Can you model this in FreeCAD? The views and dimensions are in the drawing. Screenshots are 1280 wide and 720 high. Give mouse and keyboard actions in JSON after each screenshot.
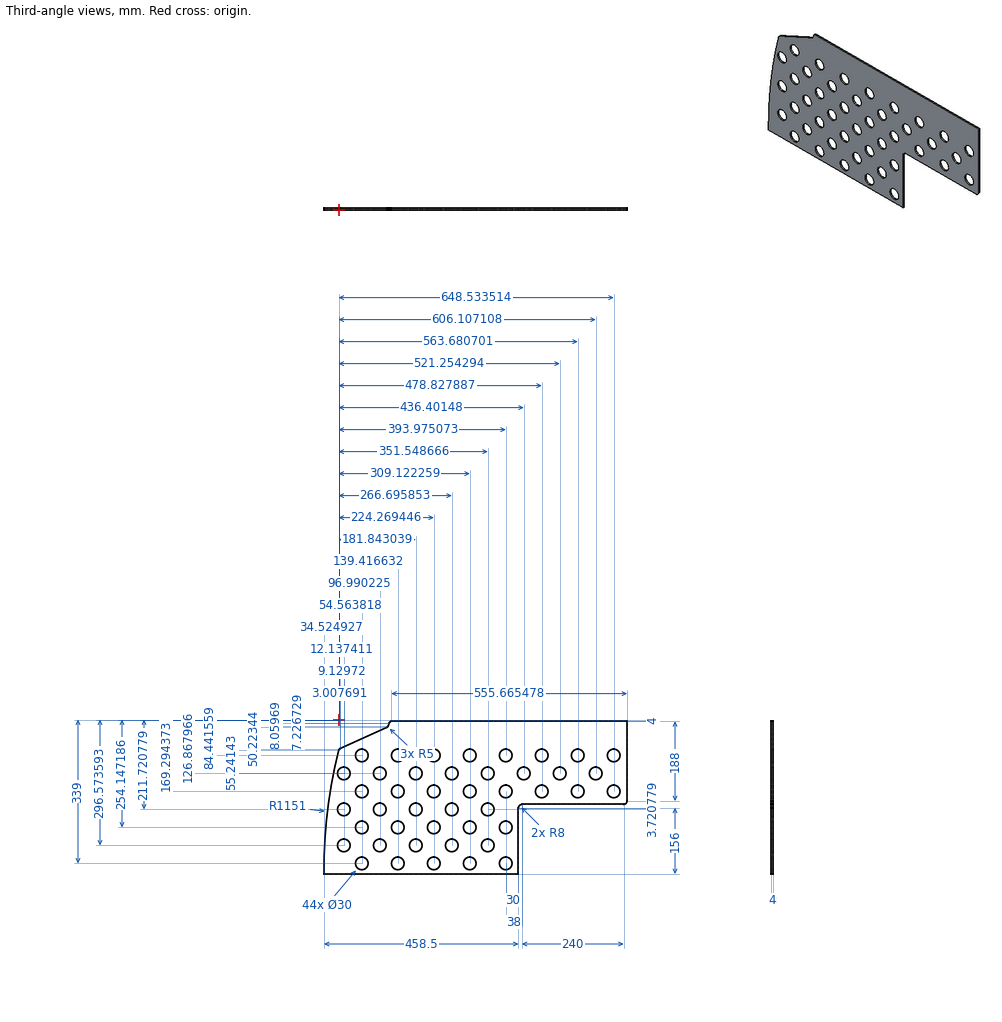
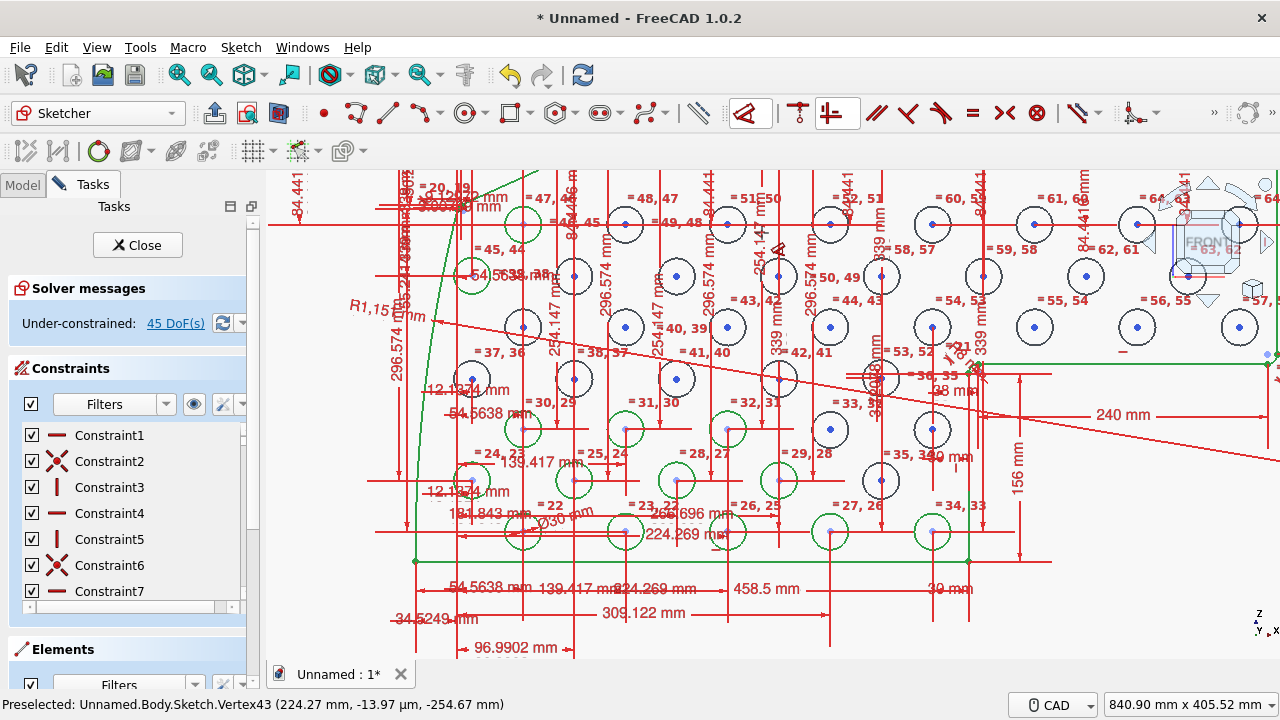
{"action": "left_click", "coordinate": [830, 430]}
{"action": "left_click", "coordinate": [644, 464]}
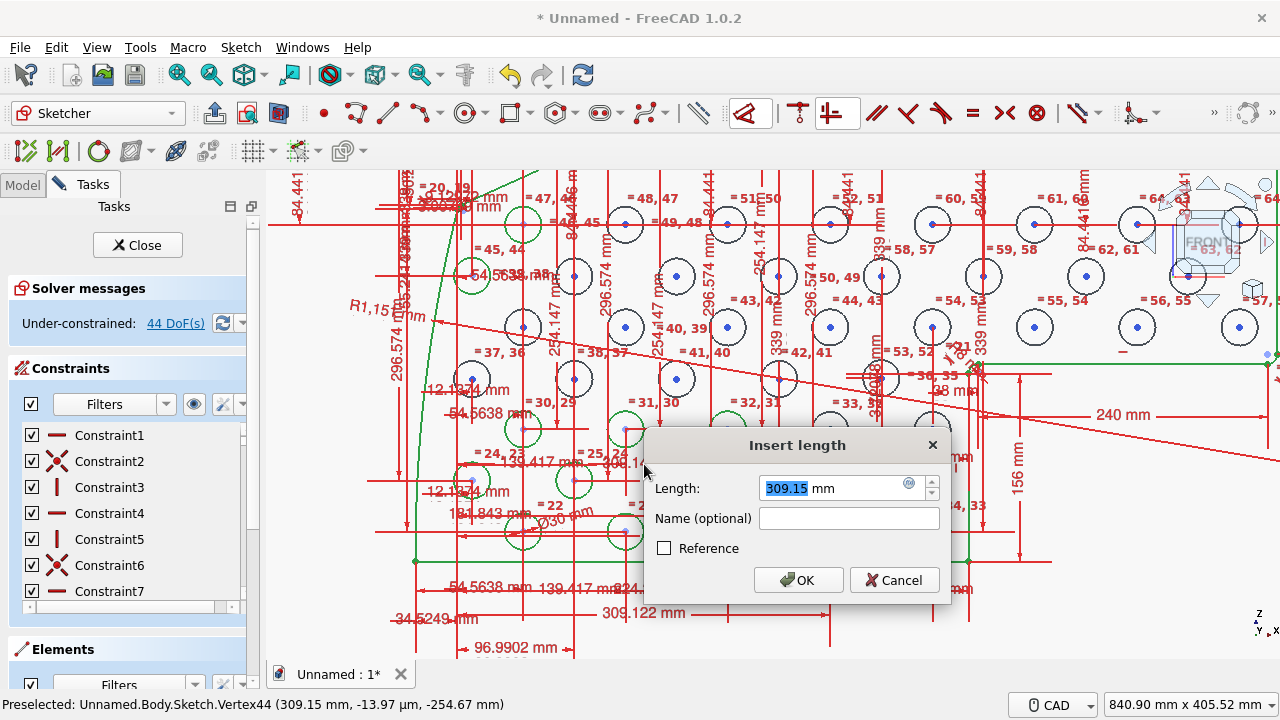
{"action": "type", "text": "309.122259"}
{"action": "key", "text": "Return"}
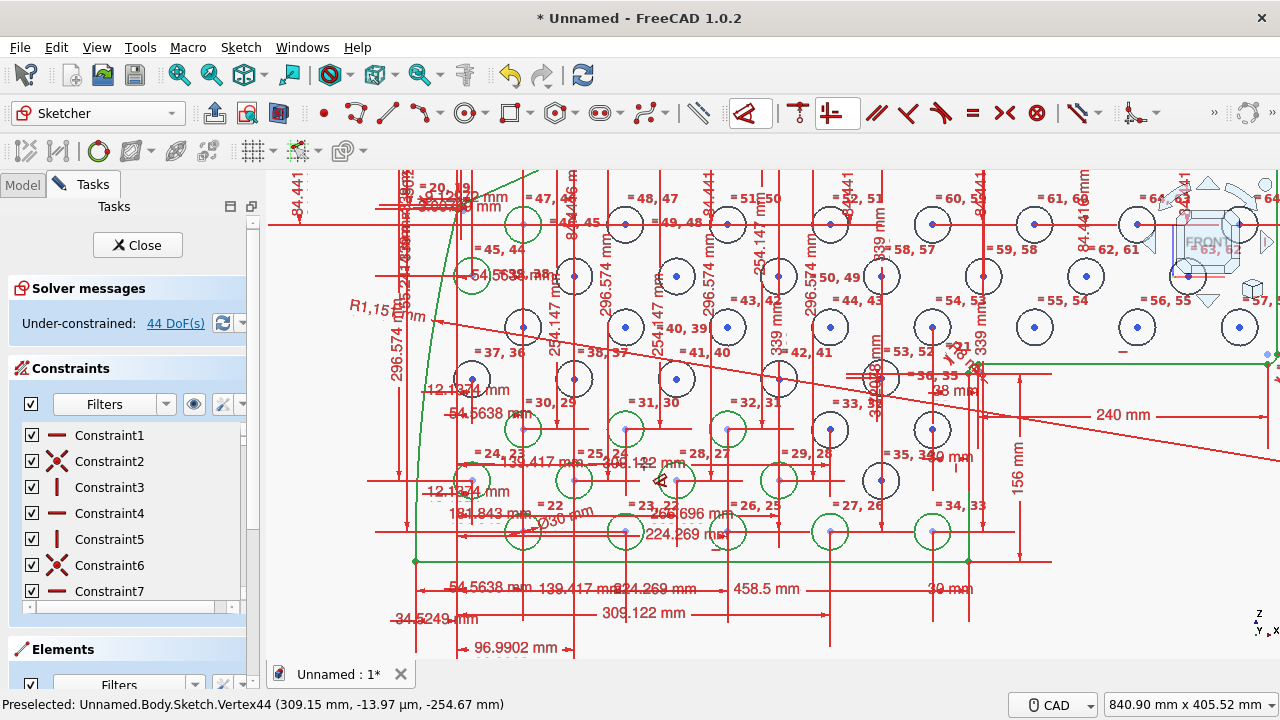
{"action": "left_click", "coordinate": [830, 430]}
{"action": "left_click", "coordinate": [864, 314]}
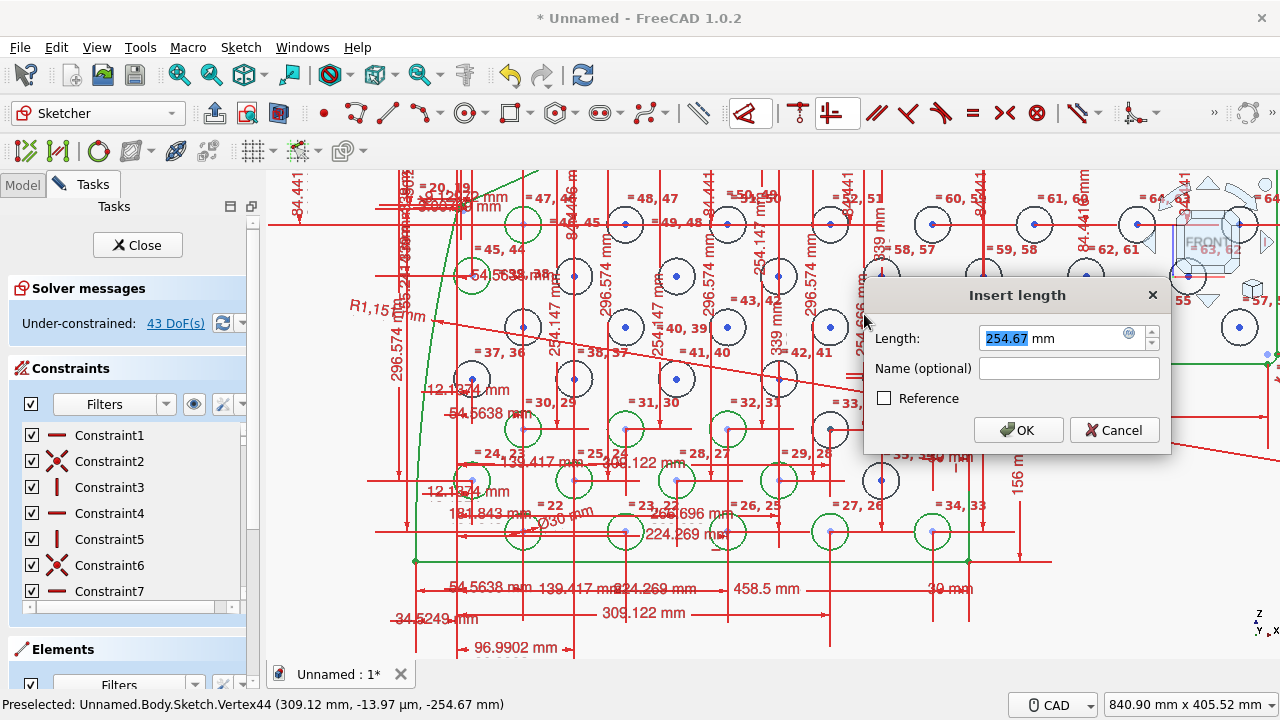
{"action": "type", "text": "254.147186"}
{"action": "key", "text": "Return"}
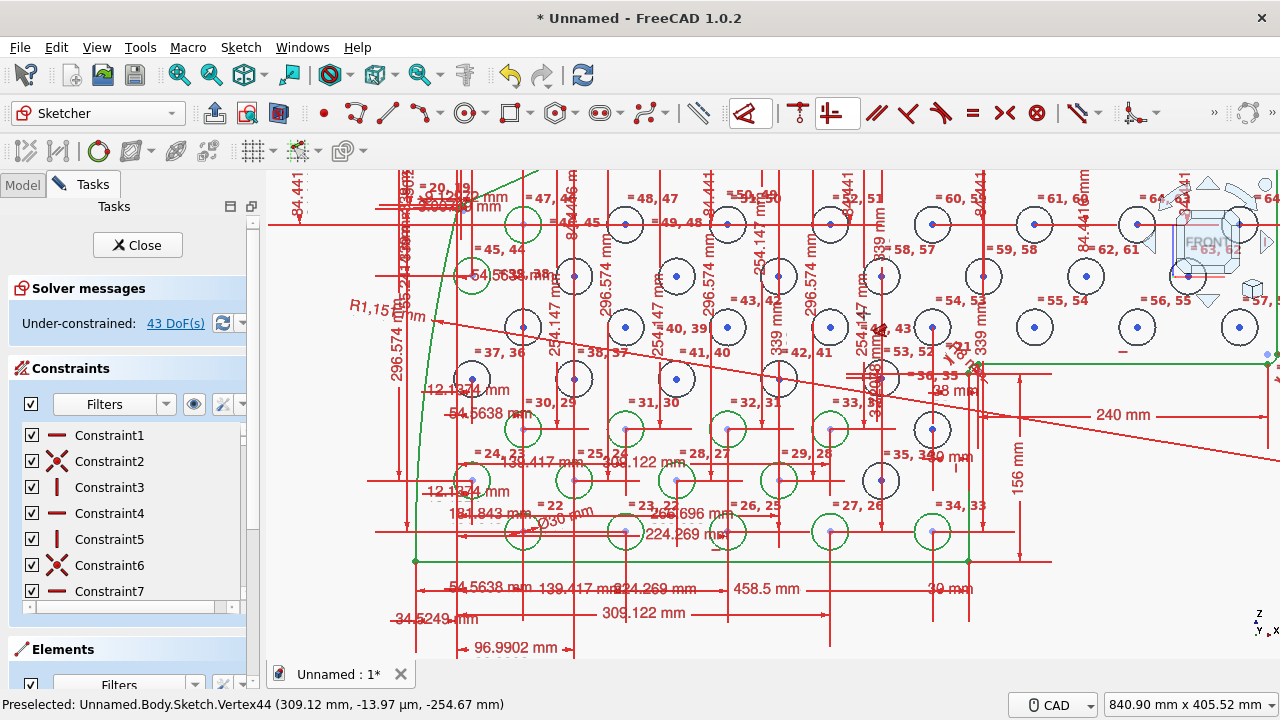
{"action": "left_click", "coordinate": [881, 481]}
{"action": "left_click", "coordinate": [767, 515]}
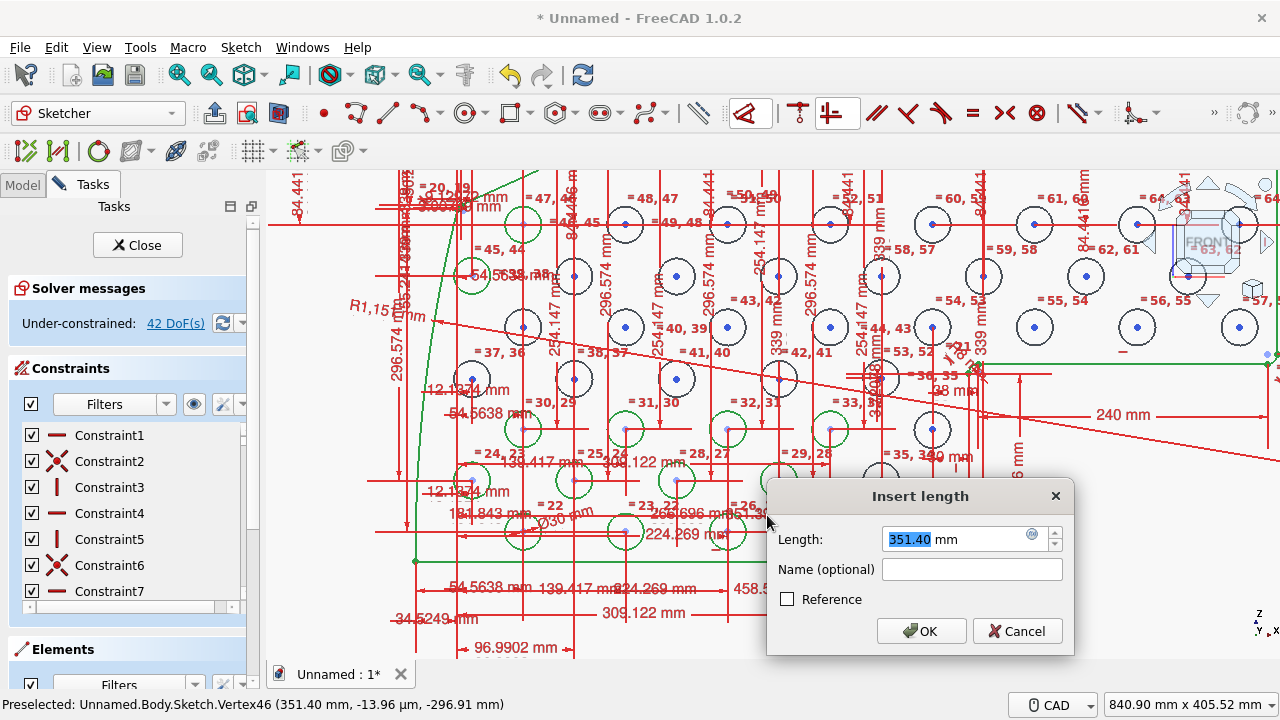
{"action": "type", "text": "351.548666"}
{"action": "key", "text": "Return"}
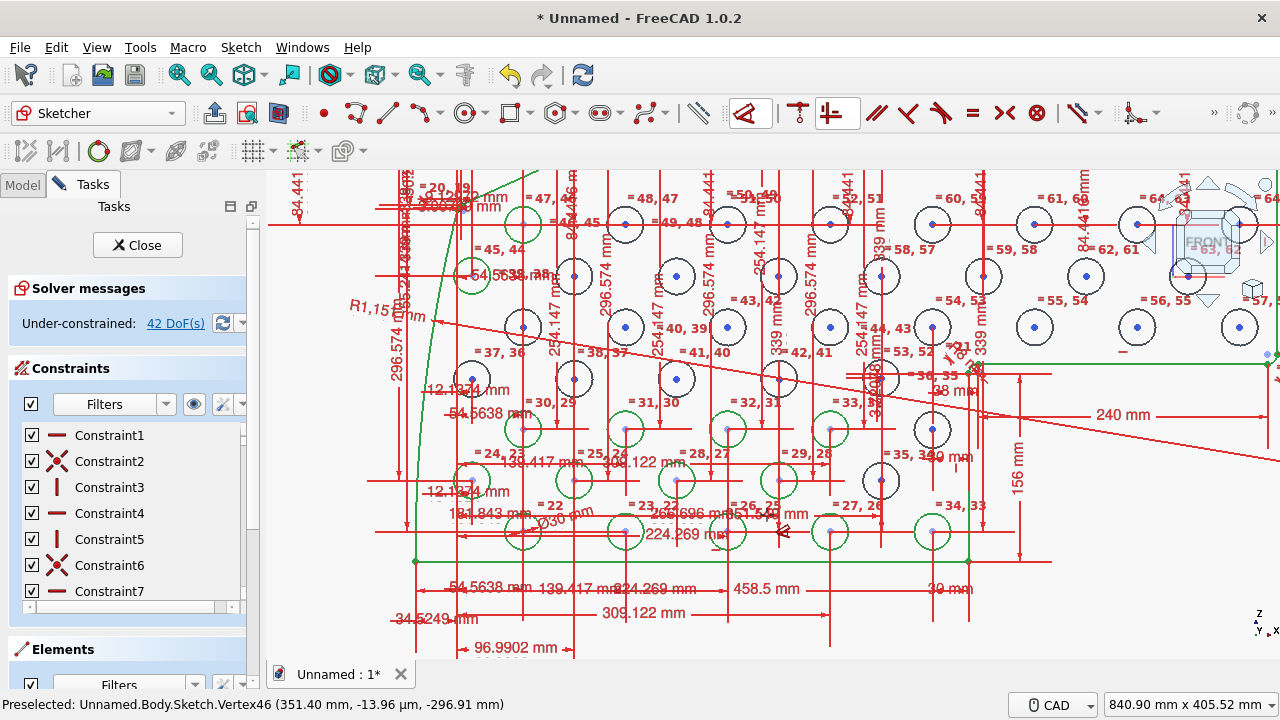
{"action": "left_click", "coordinate": [881, 481]}
{"action": "left_click", "coordinate": [915, 274]}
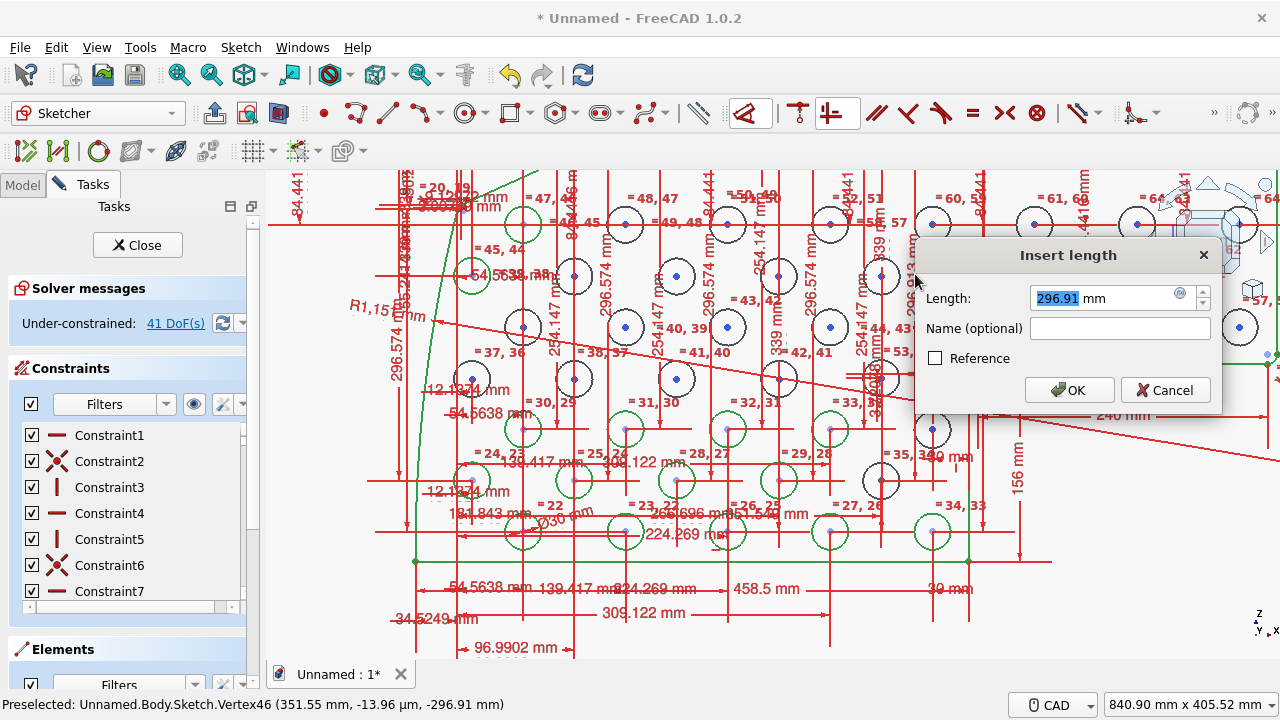
{"action": "type", "text": "296.573593"}
{"action": "key", "text": "Return"}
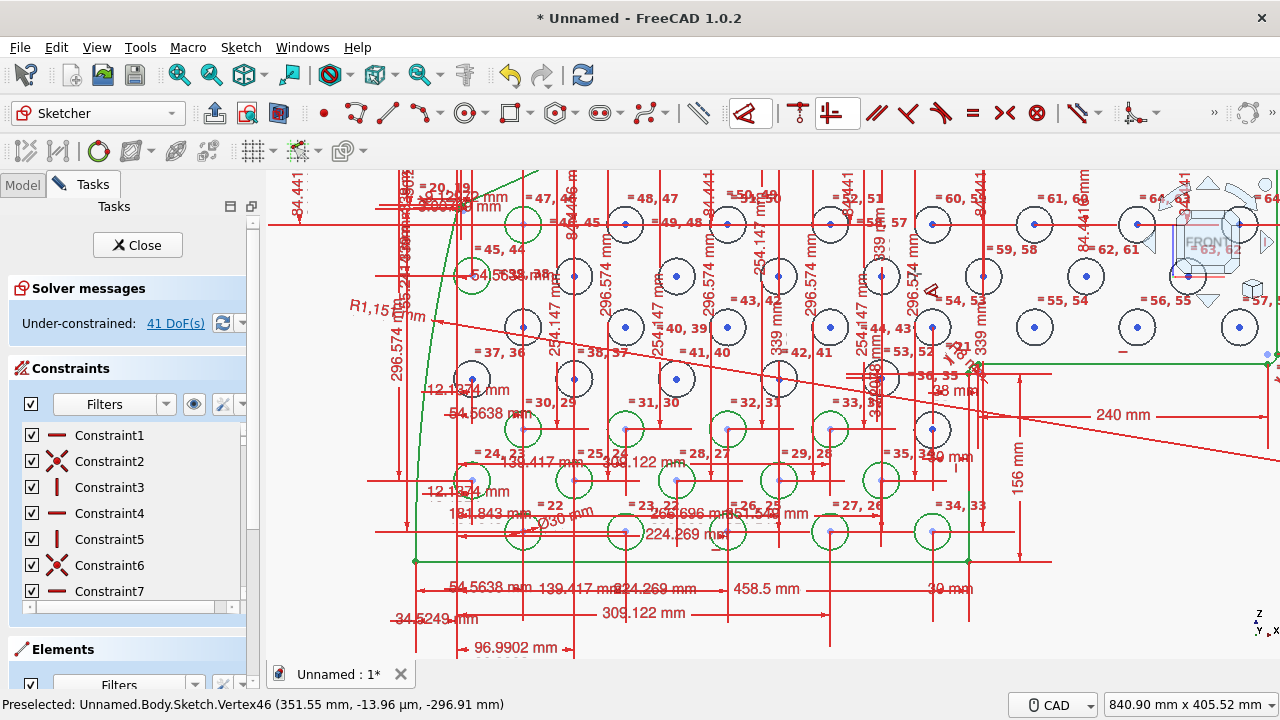
{"action": "left_click", "coordinate": [933, 430]}
{"action": "left_click", "coordinate": [967, 233]}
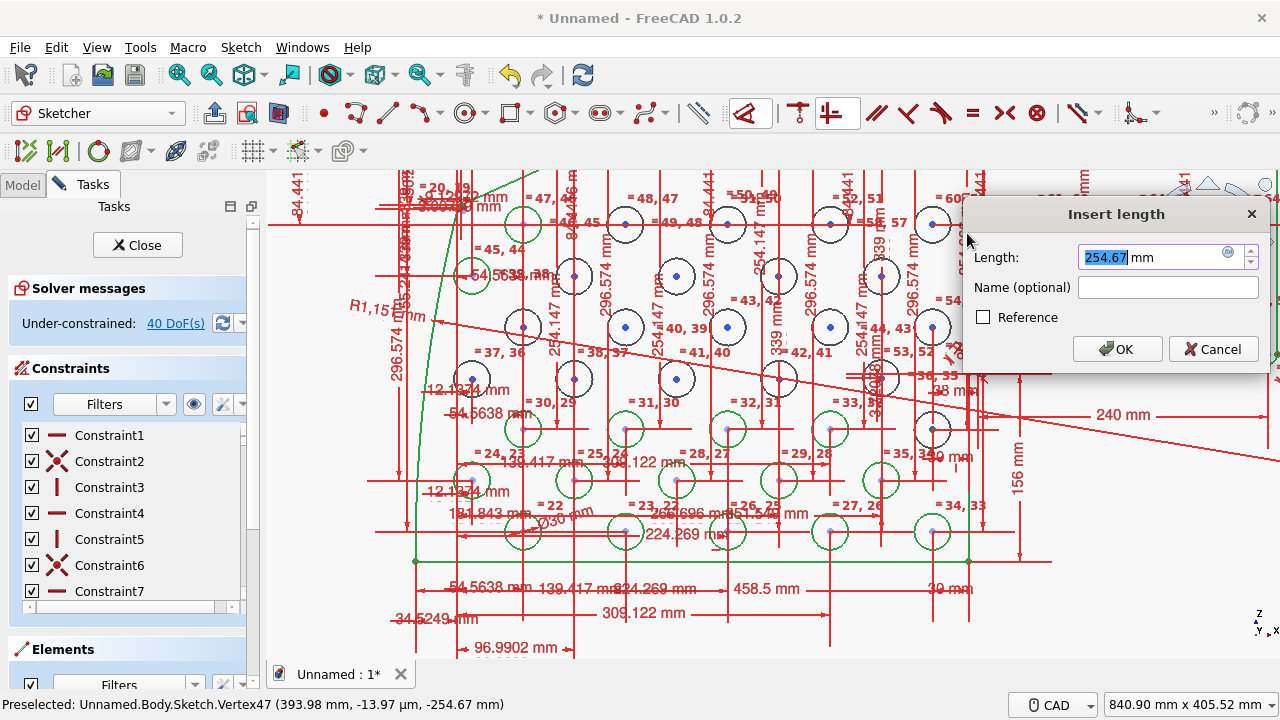
{"action": "type", "text": "254.147186"}
{"action": "key", "text": "Return"}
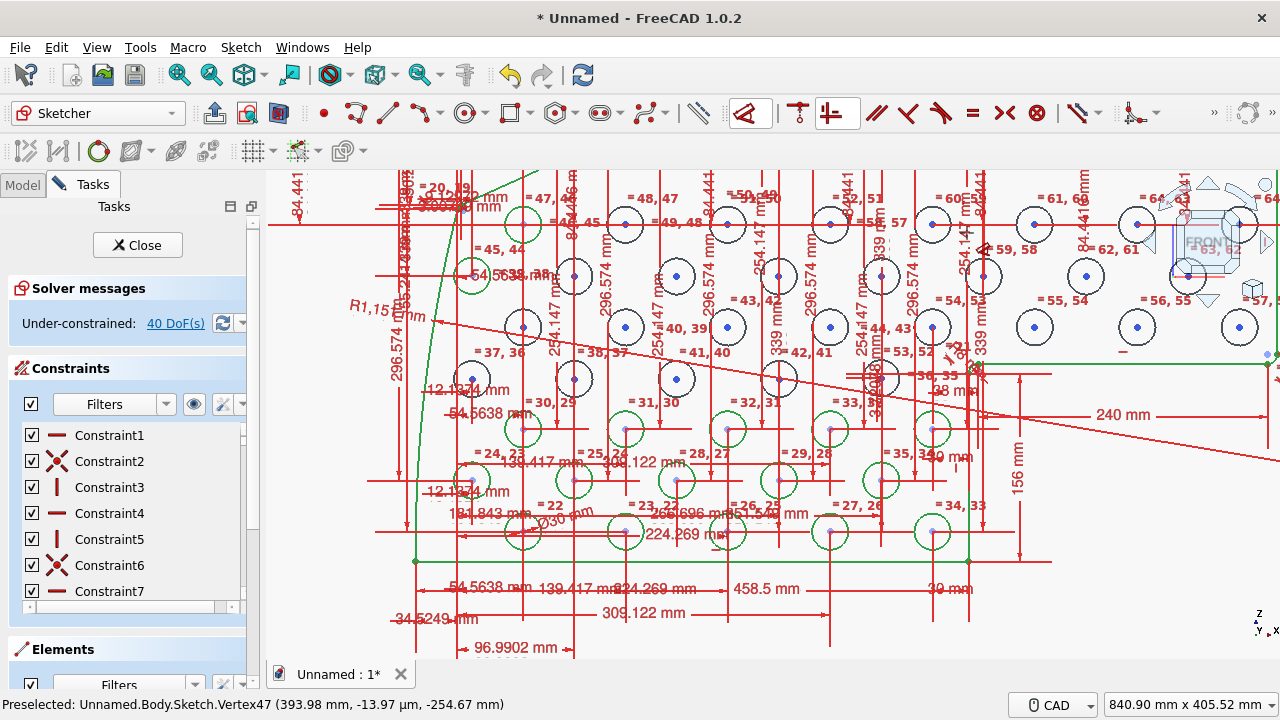
{"action": "left_click", "coordinate": [472, 379]}
{"action": "left_click", "coordinate": [554, 247]}